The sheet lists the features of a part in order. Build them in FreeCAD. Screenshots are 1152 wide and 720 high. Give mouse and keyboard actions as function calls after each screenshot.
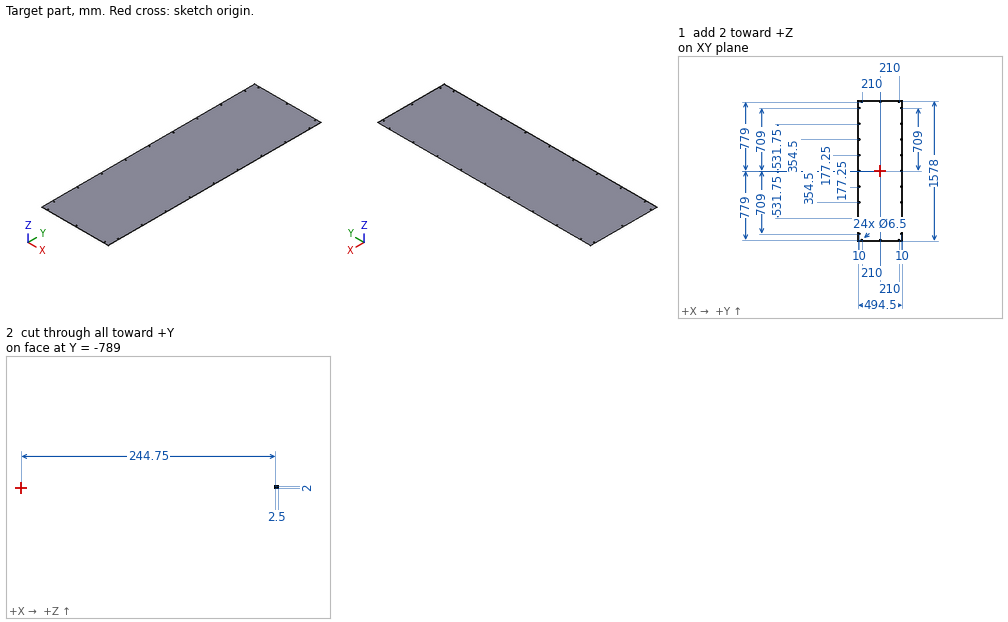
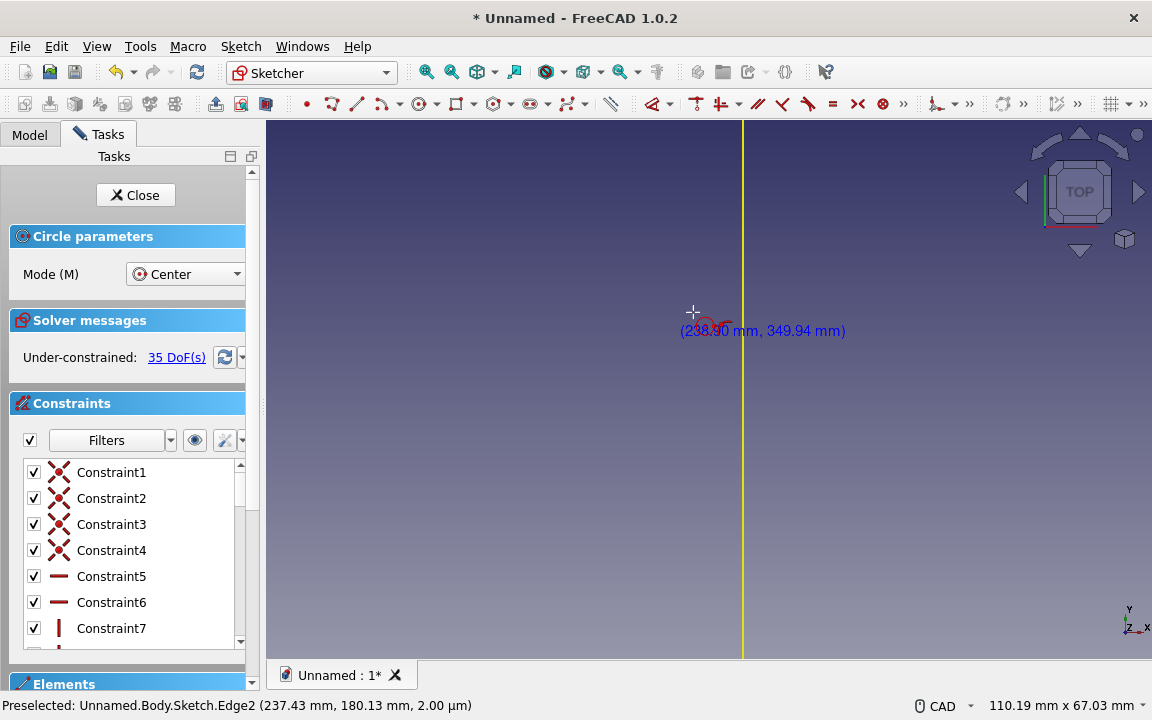
scroll(706, 294, down, 17)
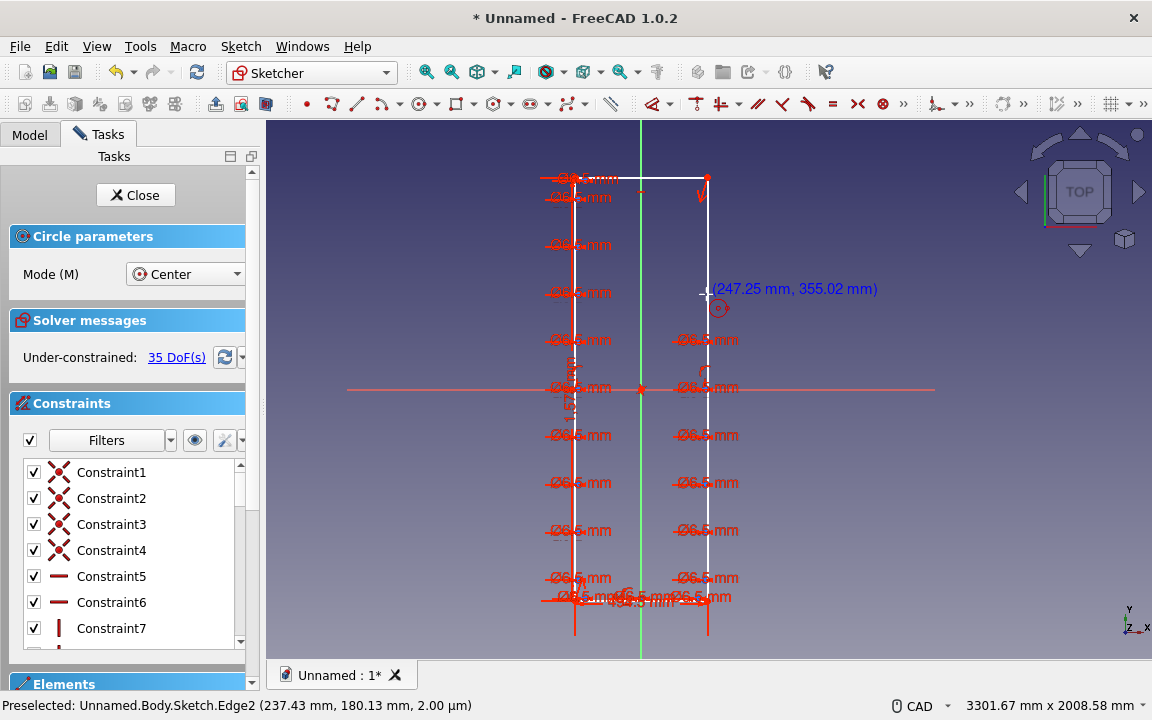
scroll(705, 294, up, 9)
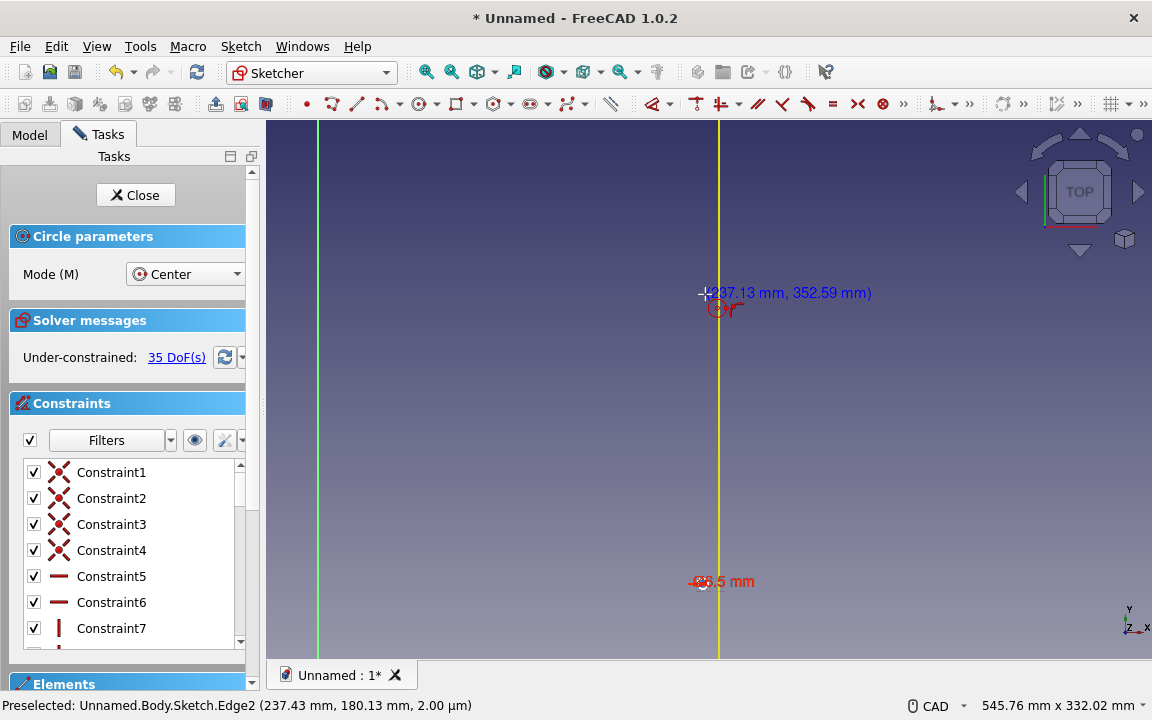
click(703, 295)
move(699, 292)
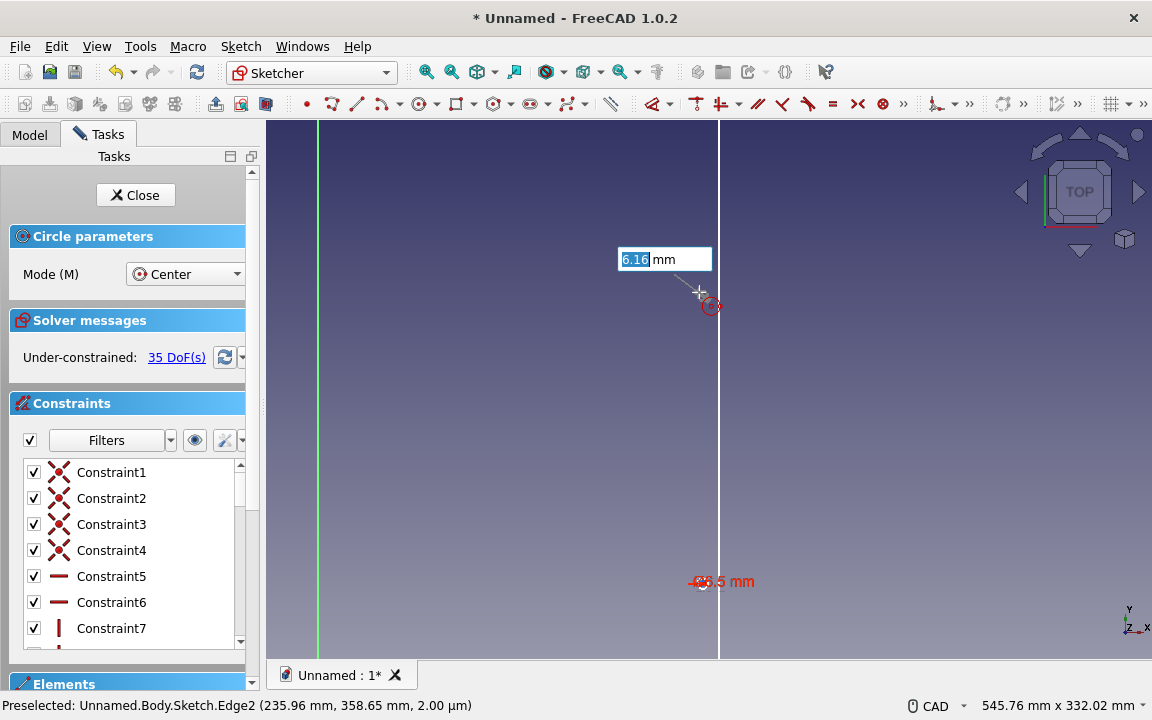
text(6.5)
key(Return)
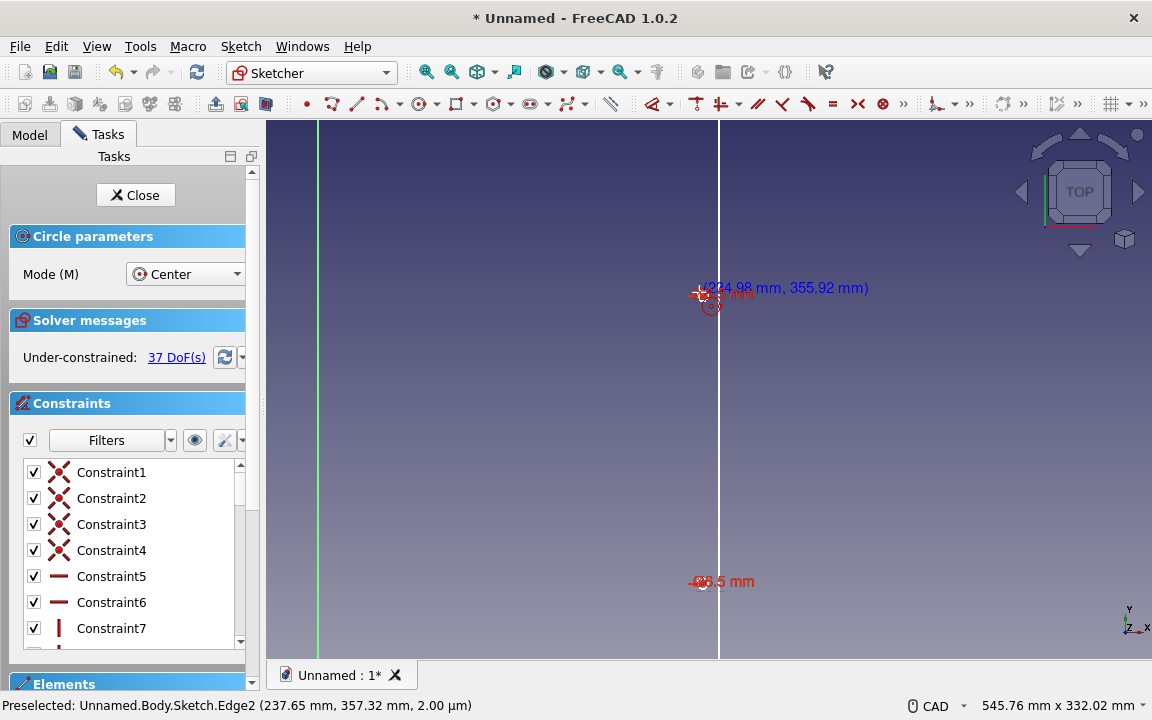
scroll(691, 314, down, 10)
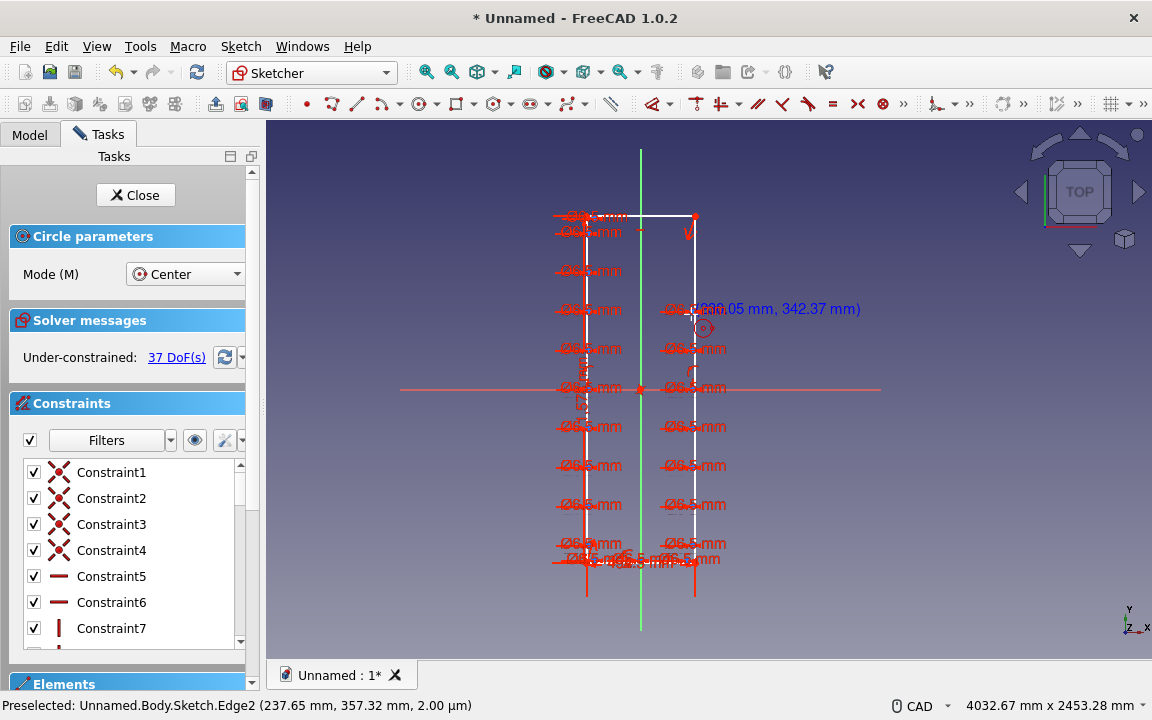
scroll(641, 219, up, 18)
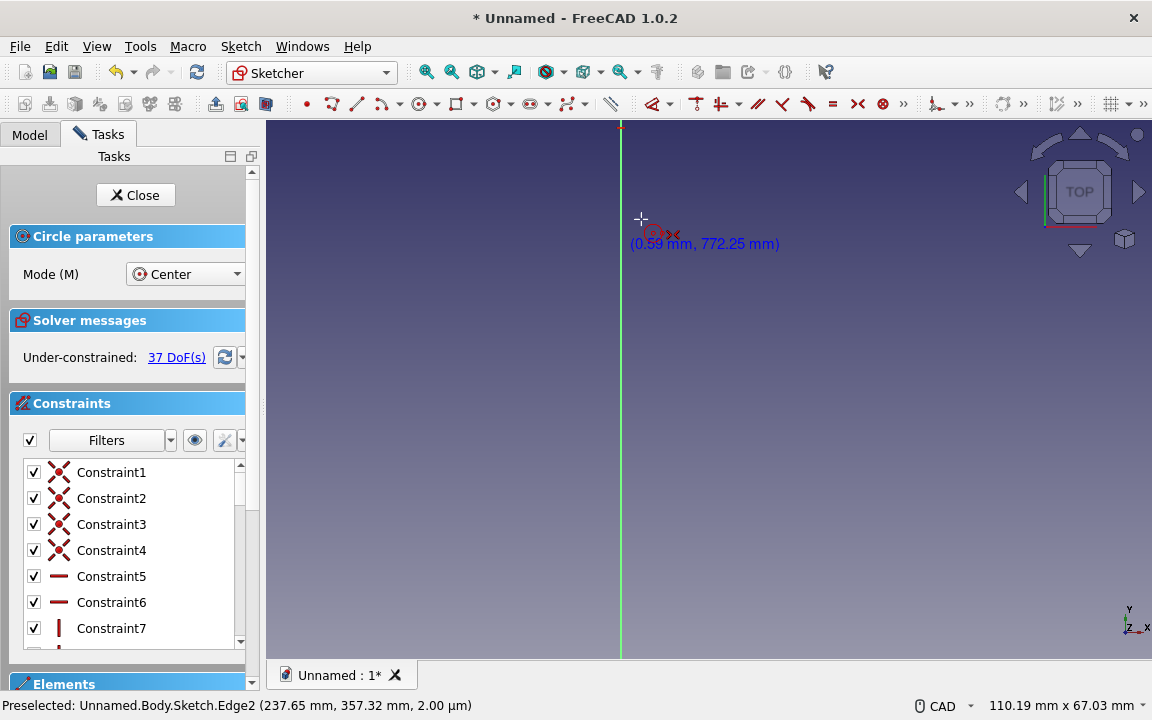
scroll(641, 180, down, 17)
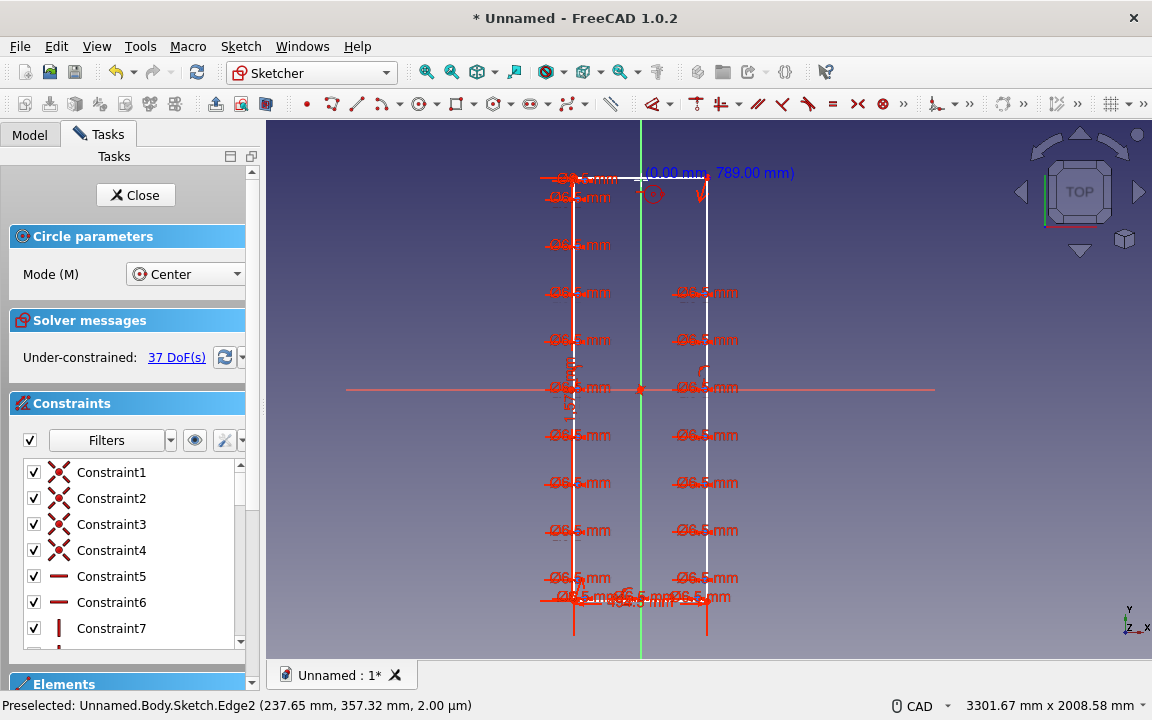
scroll(641, 181, up, 9)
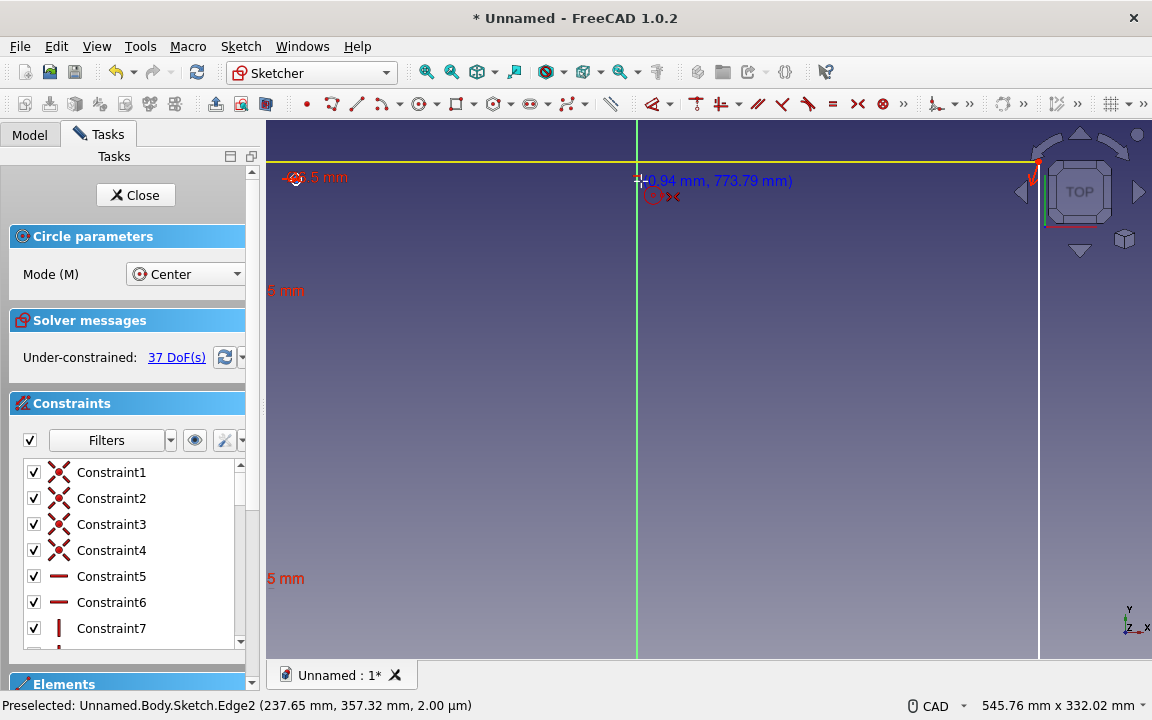
click(637, 178)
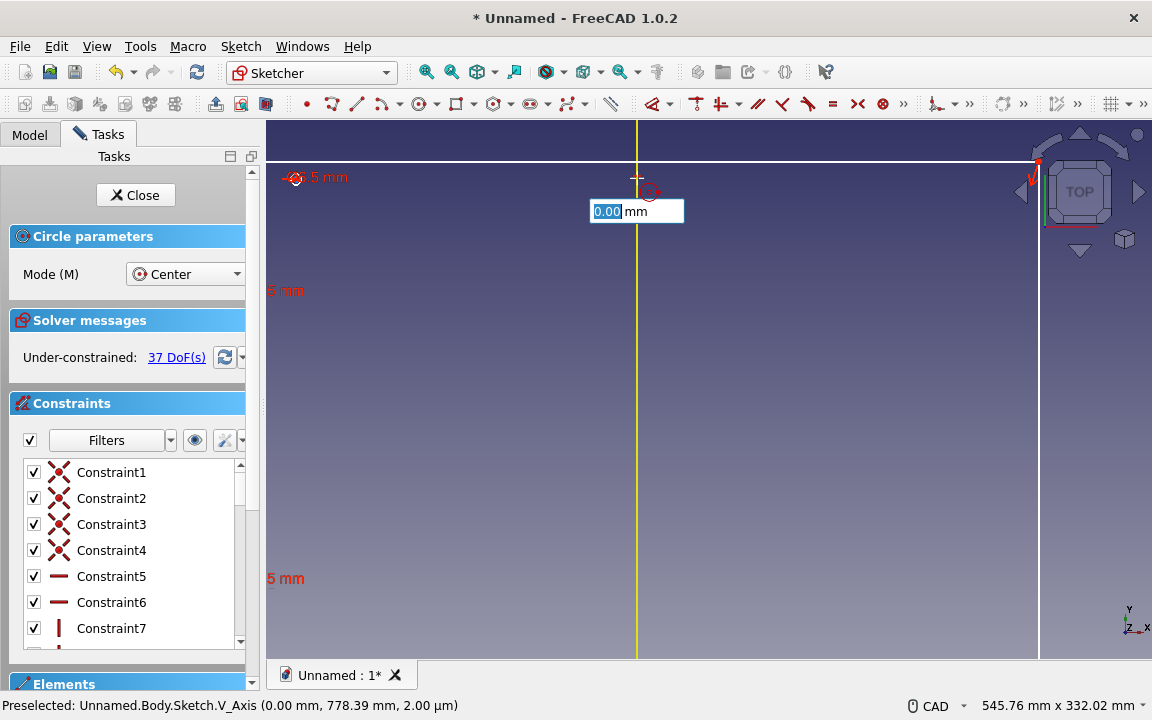
scroll(642, 176, up, 6)
move(642, 176)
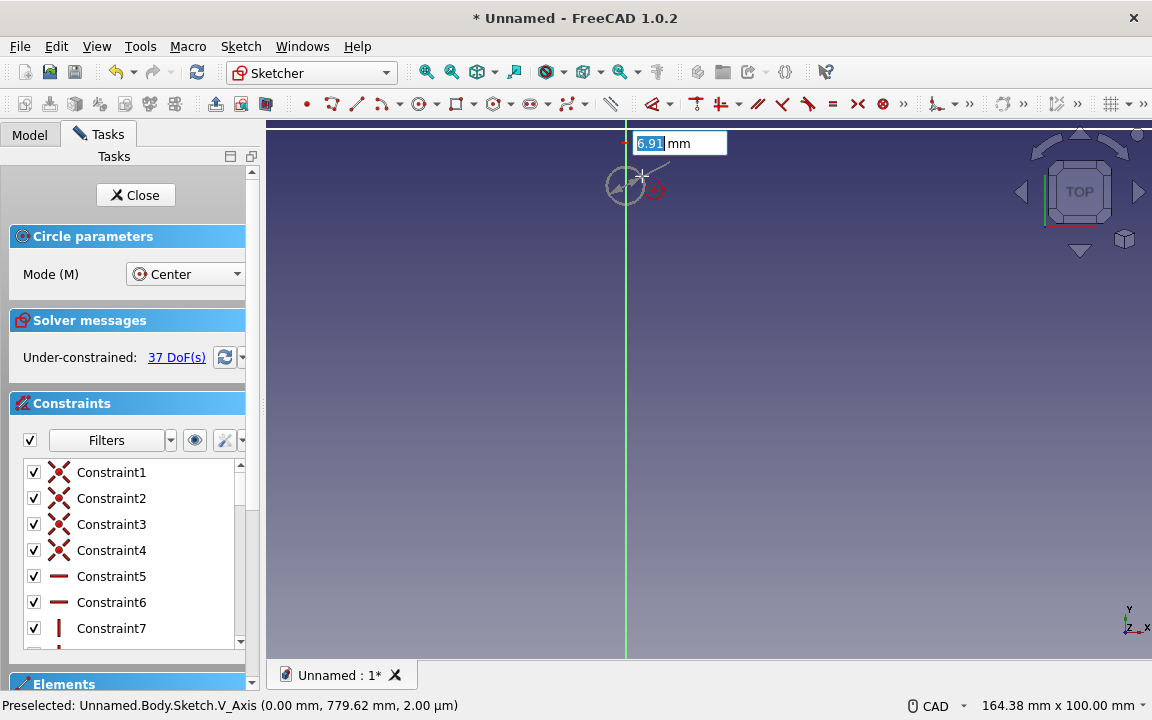
text(6.5)
key(Return)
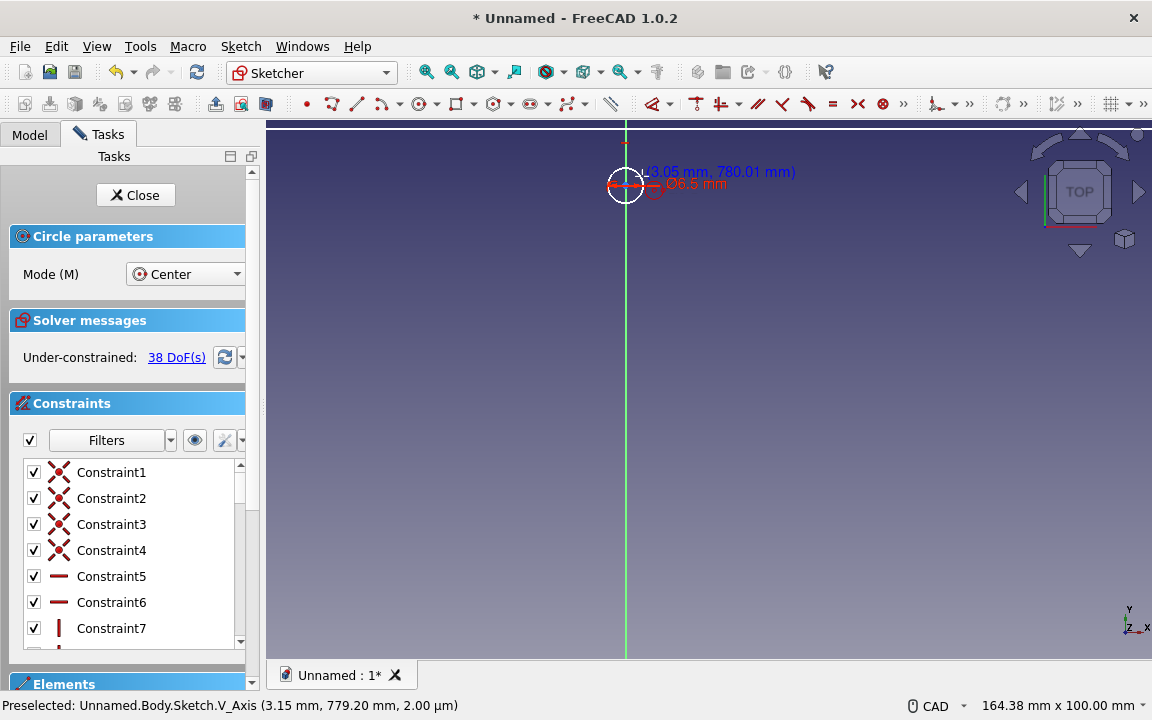
scroll(641, 180, down, 15)